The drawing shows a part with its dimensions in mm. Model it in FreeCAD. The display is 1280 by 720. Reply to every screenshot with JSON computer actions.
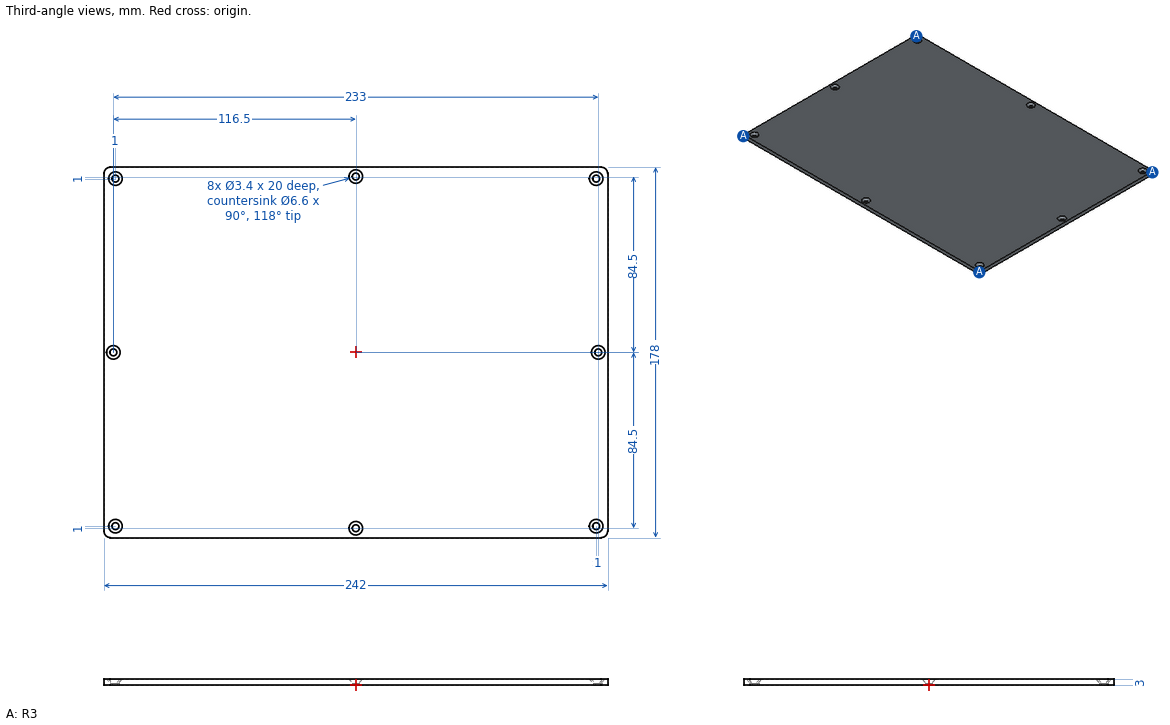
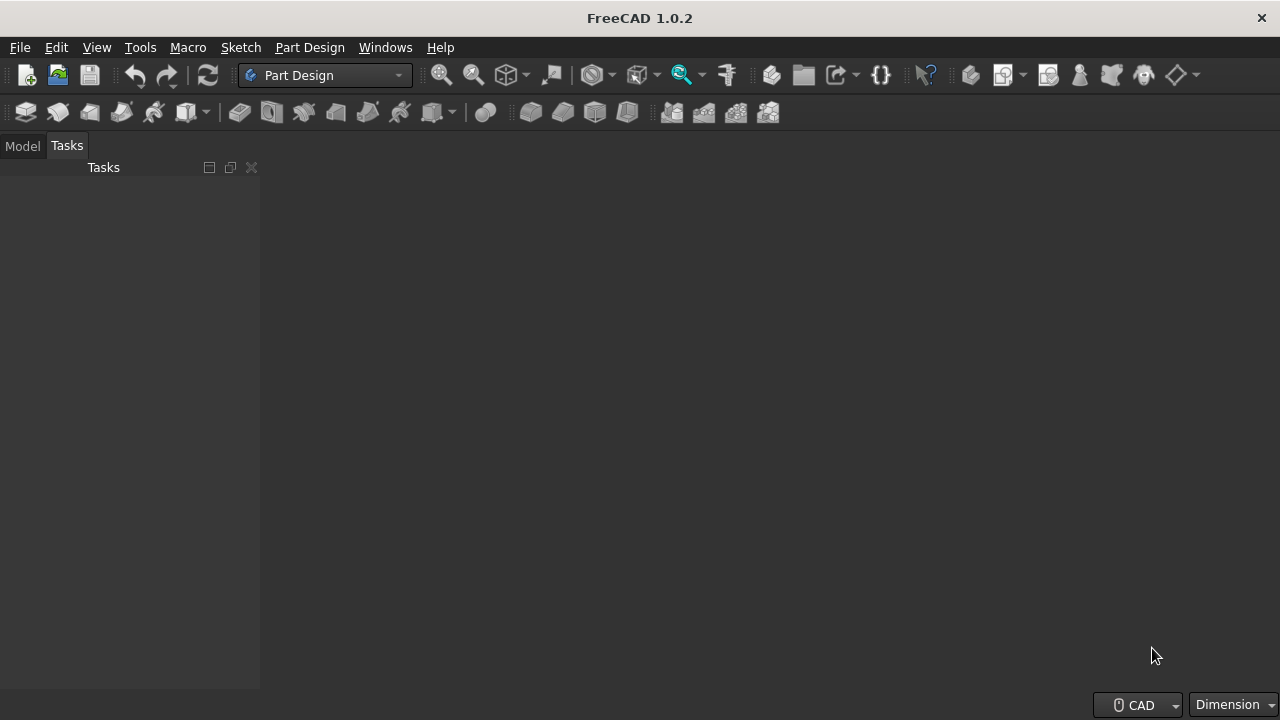
{"action": "left_click", "coordinate": [26, 76]}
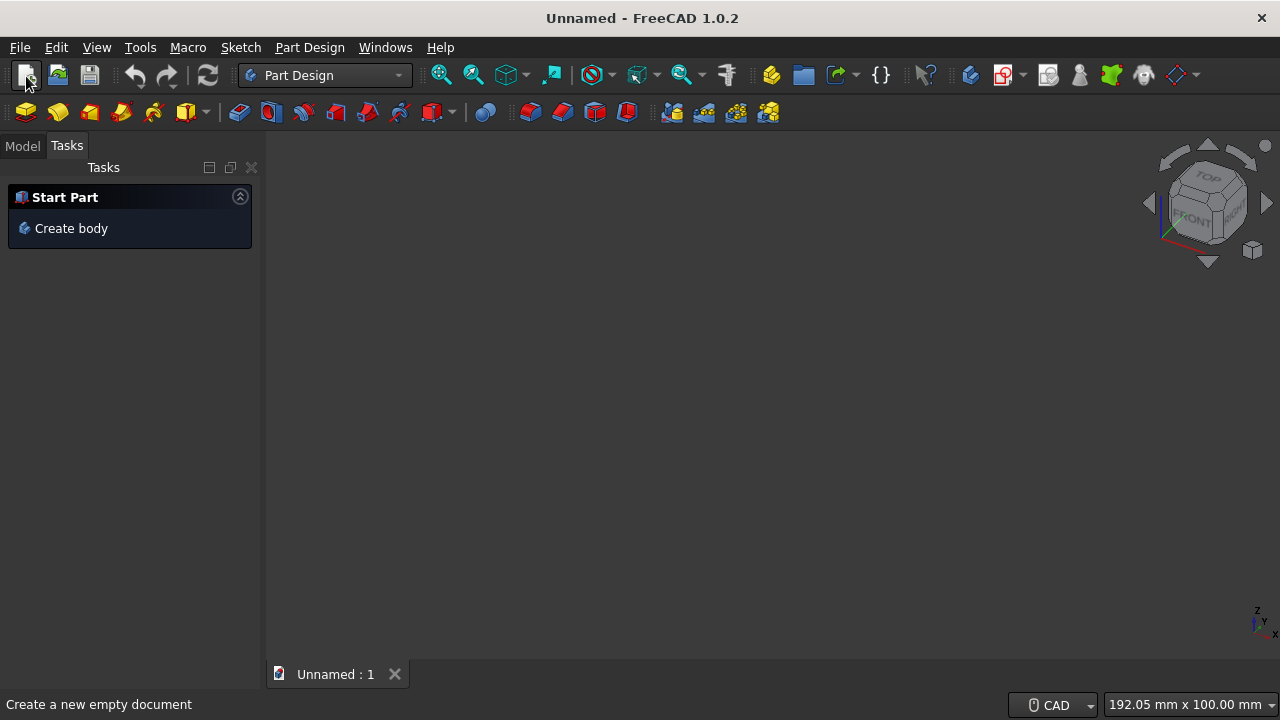
{"action": "left_click", "coordinate": [1004, 76]}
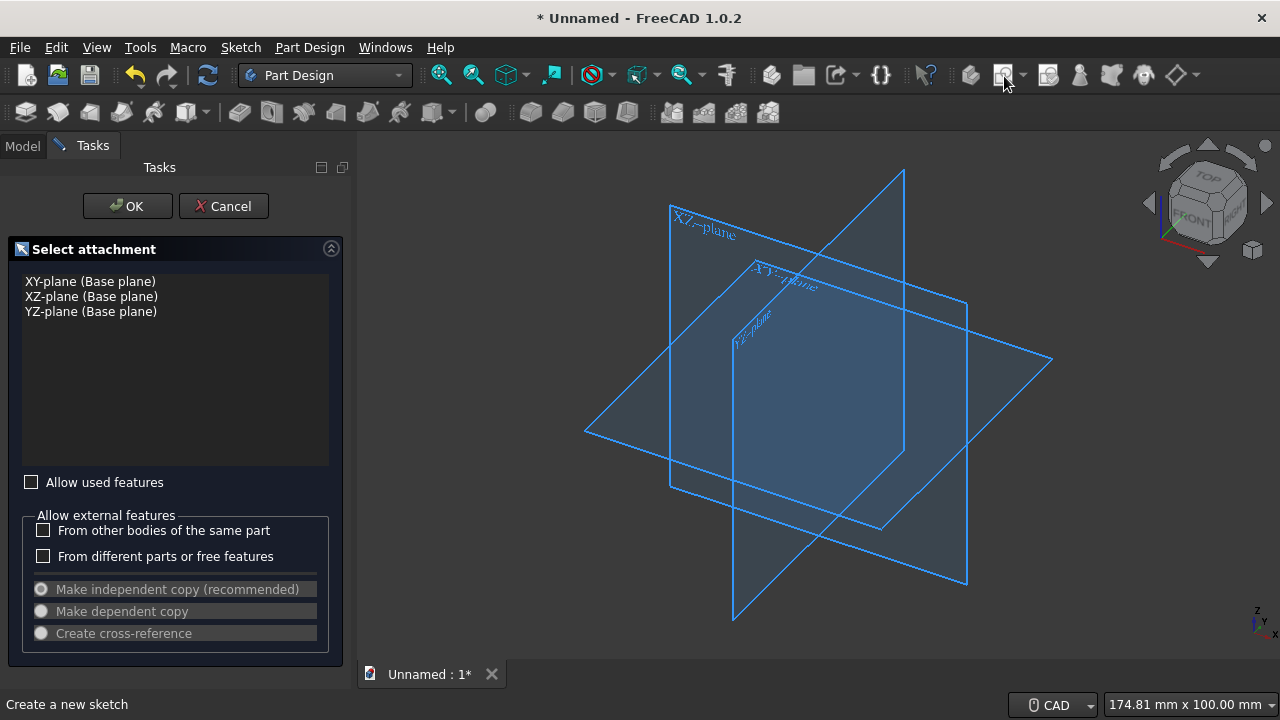
{"action": "left_click", "coordinate": [82, 282]}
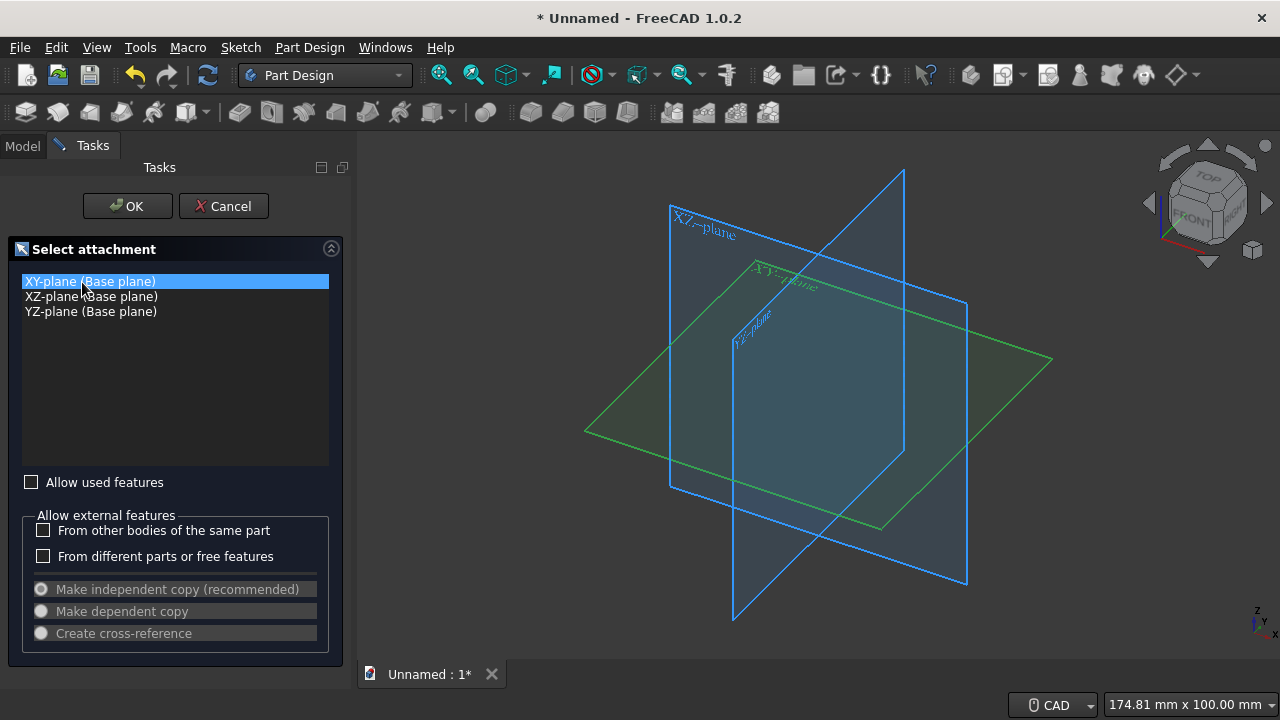
{"action": "left_click", "coordinate": [128, 206]}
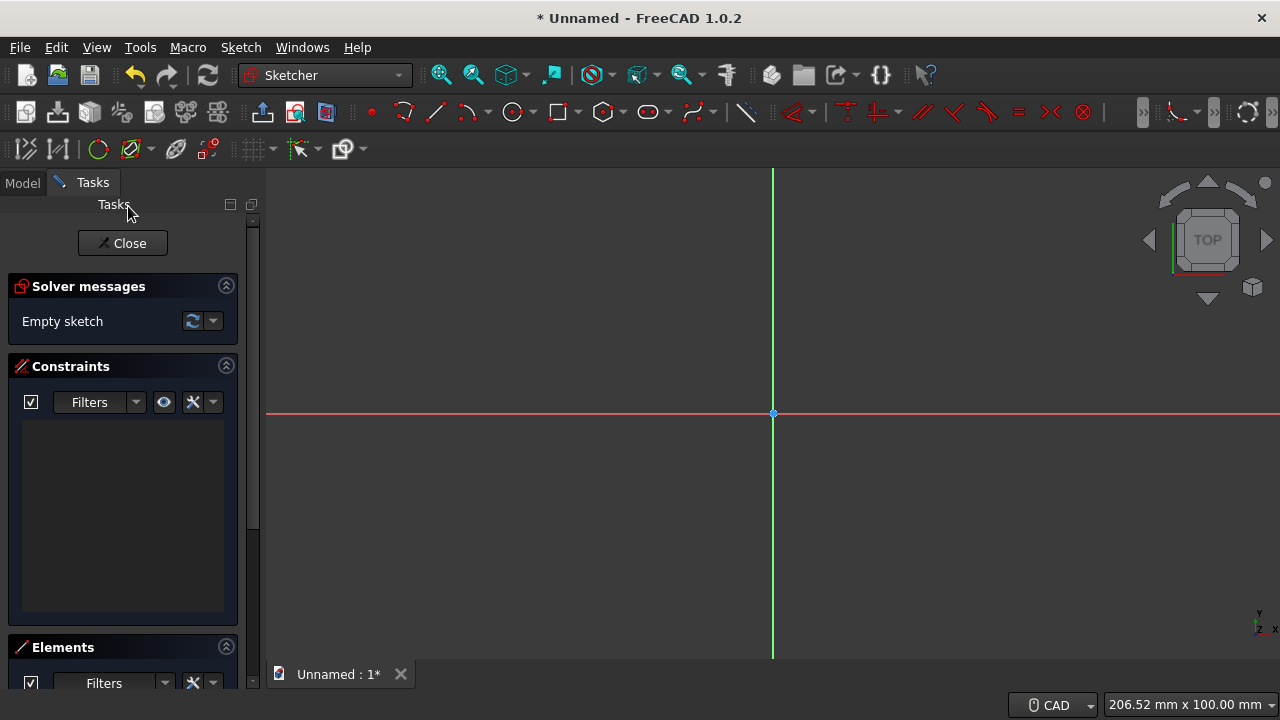
{"action": "scroll", "coordinate": [665, 414], "scroll_direction": "down", "scroll_amount": 5}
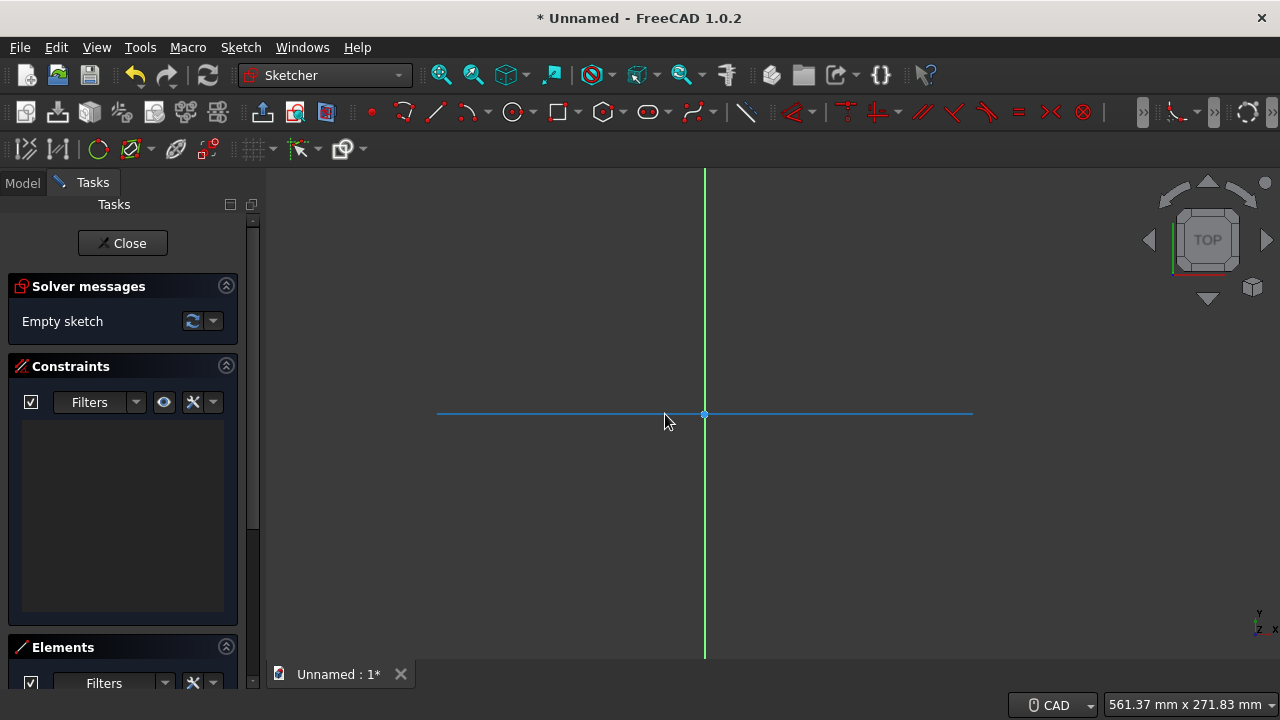
{"action": "left_click", "coordinate": [580, 112]}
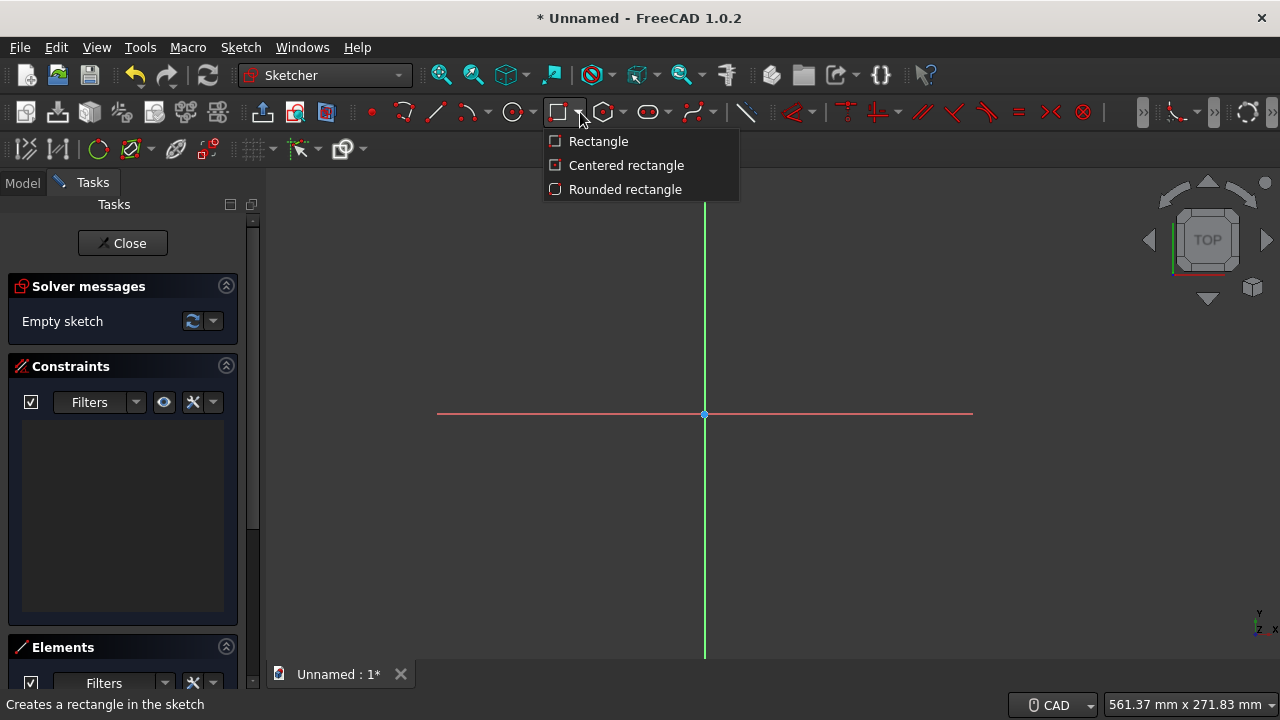
{"action": "left_click", "coordinate": [642, 165]}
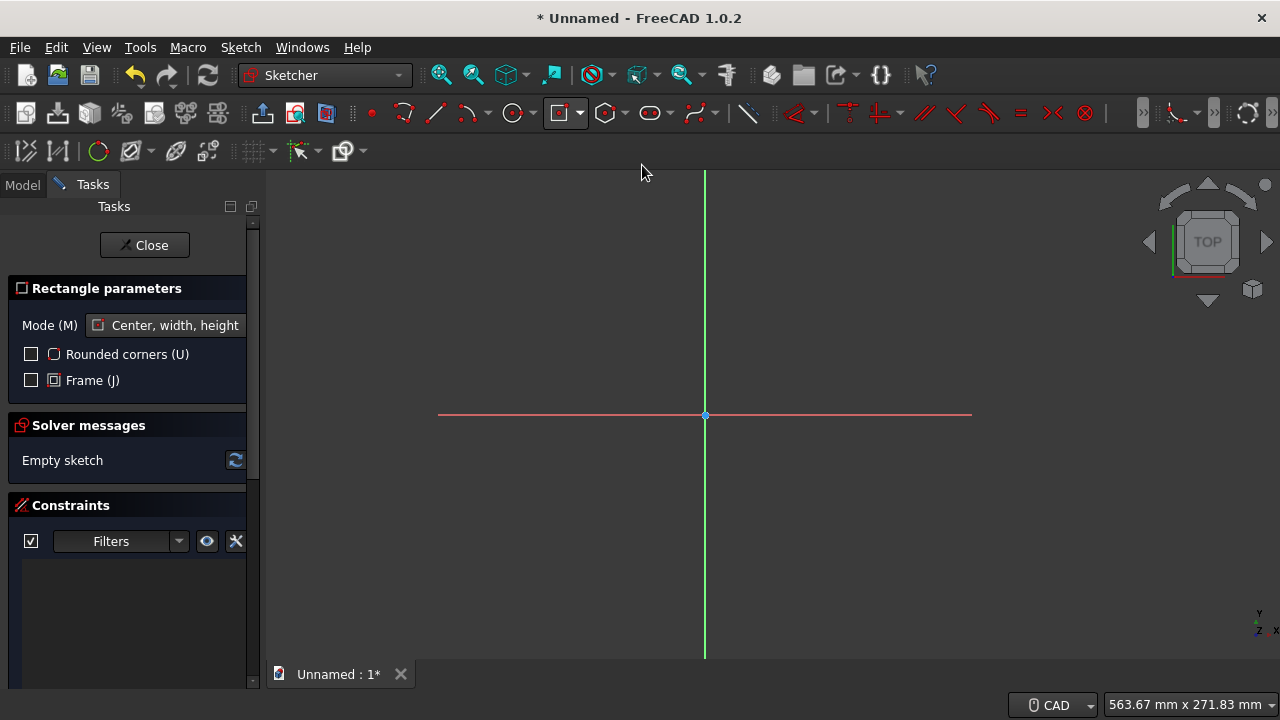
{"action": "left_click", "coordinate": [705, 415]}
{"action": "left_click", "coordinate": [923, 255]}
{"action": "key", "text": "Escape"}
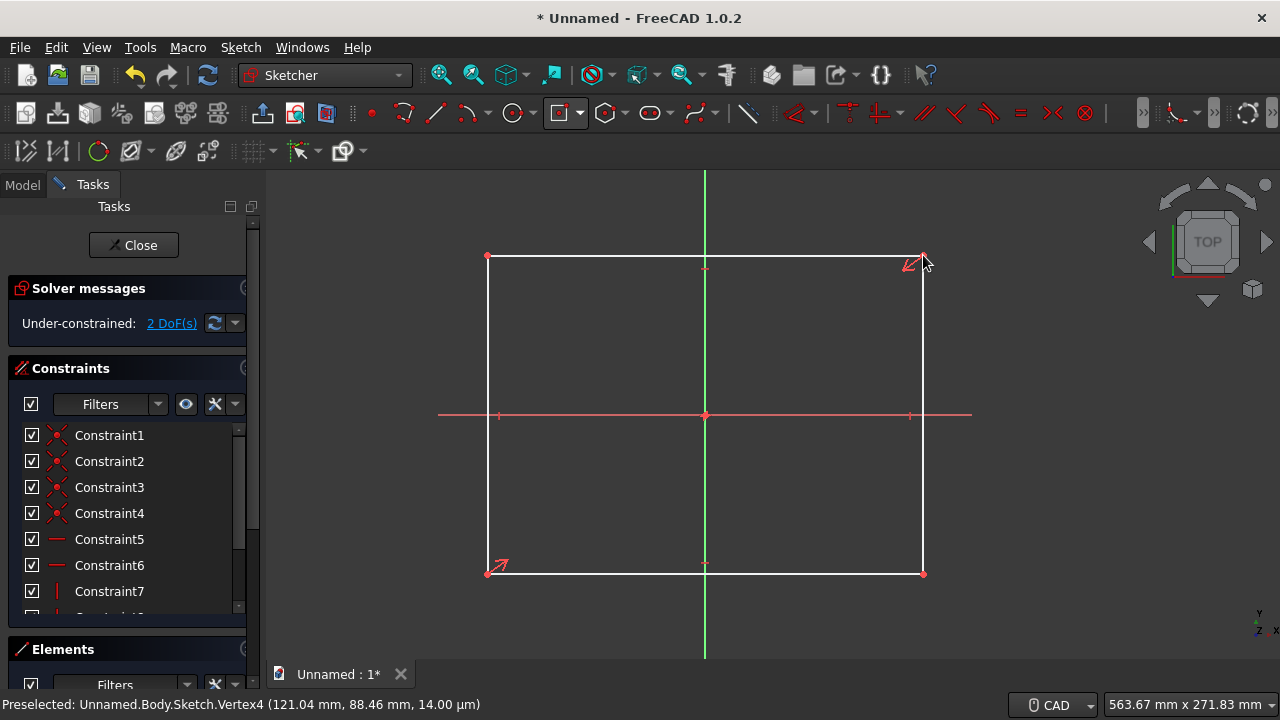
{"action": "left_click", "coordinate": [618, 574]}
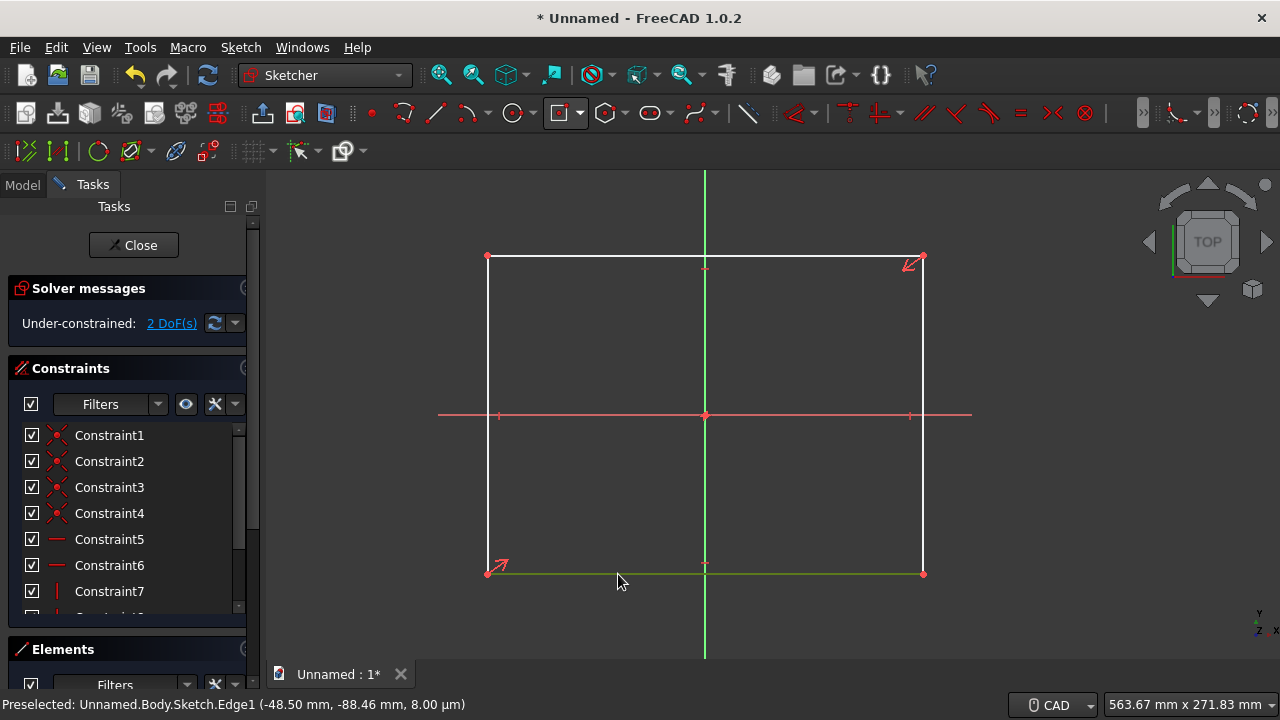
{"action": "key", "text": "l"}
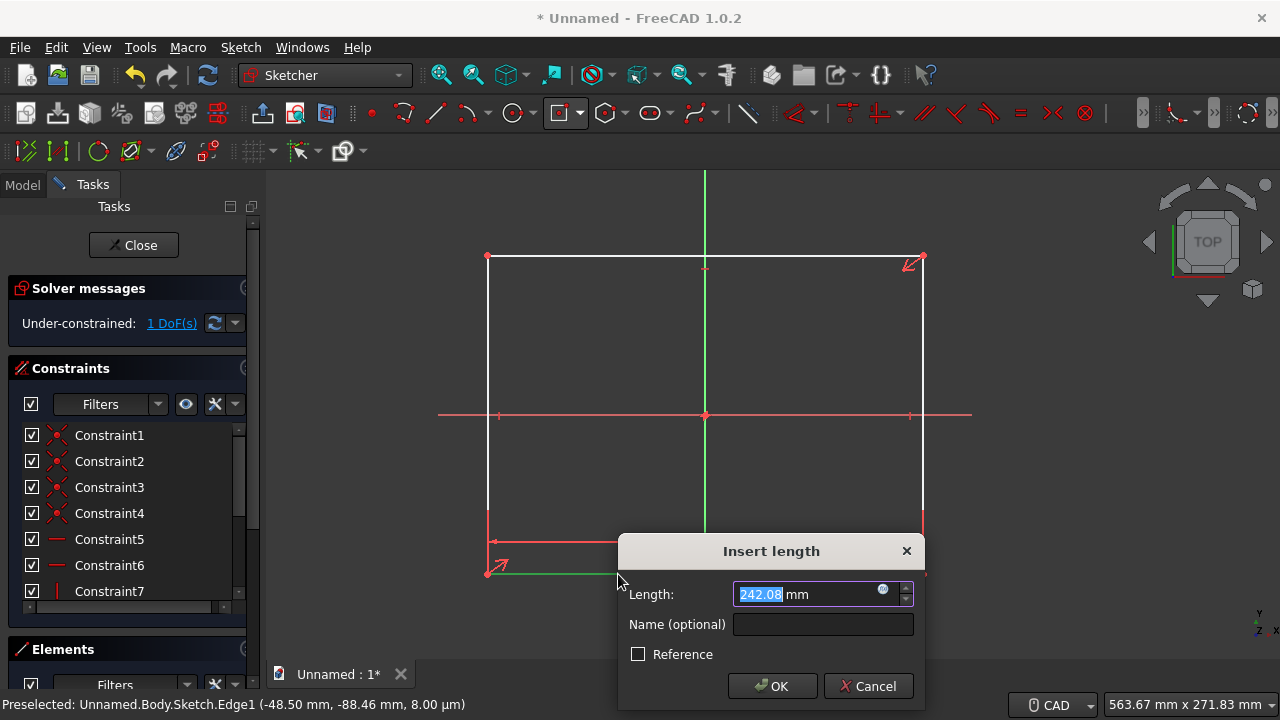
{"action": "type", "text": "242"}
{"action": "key", "text": "Return"}